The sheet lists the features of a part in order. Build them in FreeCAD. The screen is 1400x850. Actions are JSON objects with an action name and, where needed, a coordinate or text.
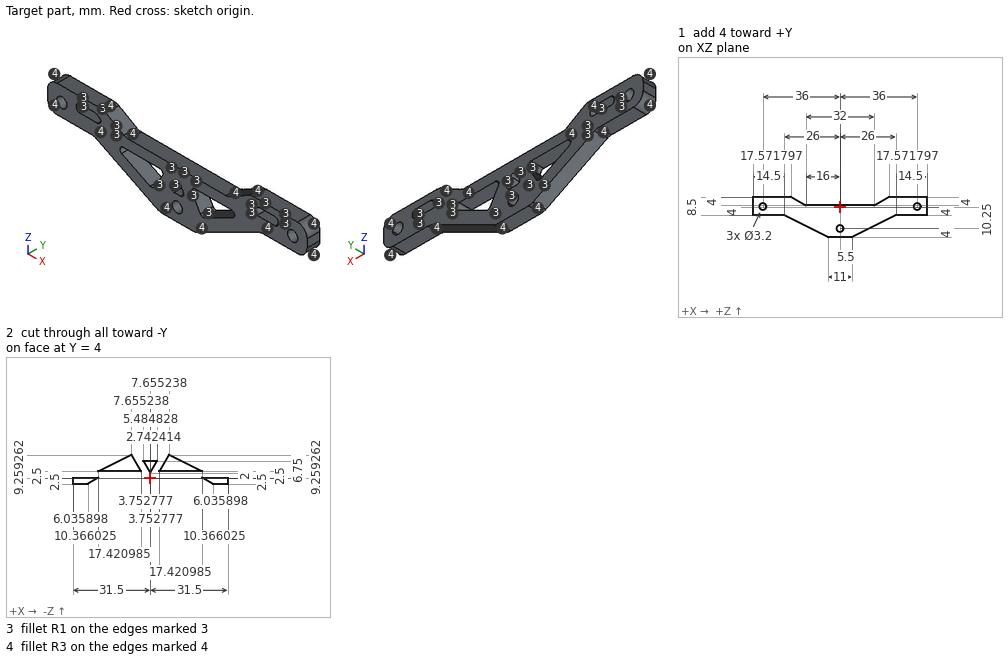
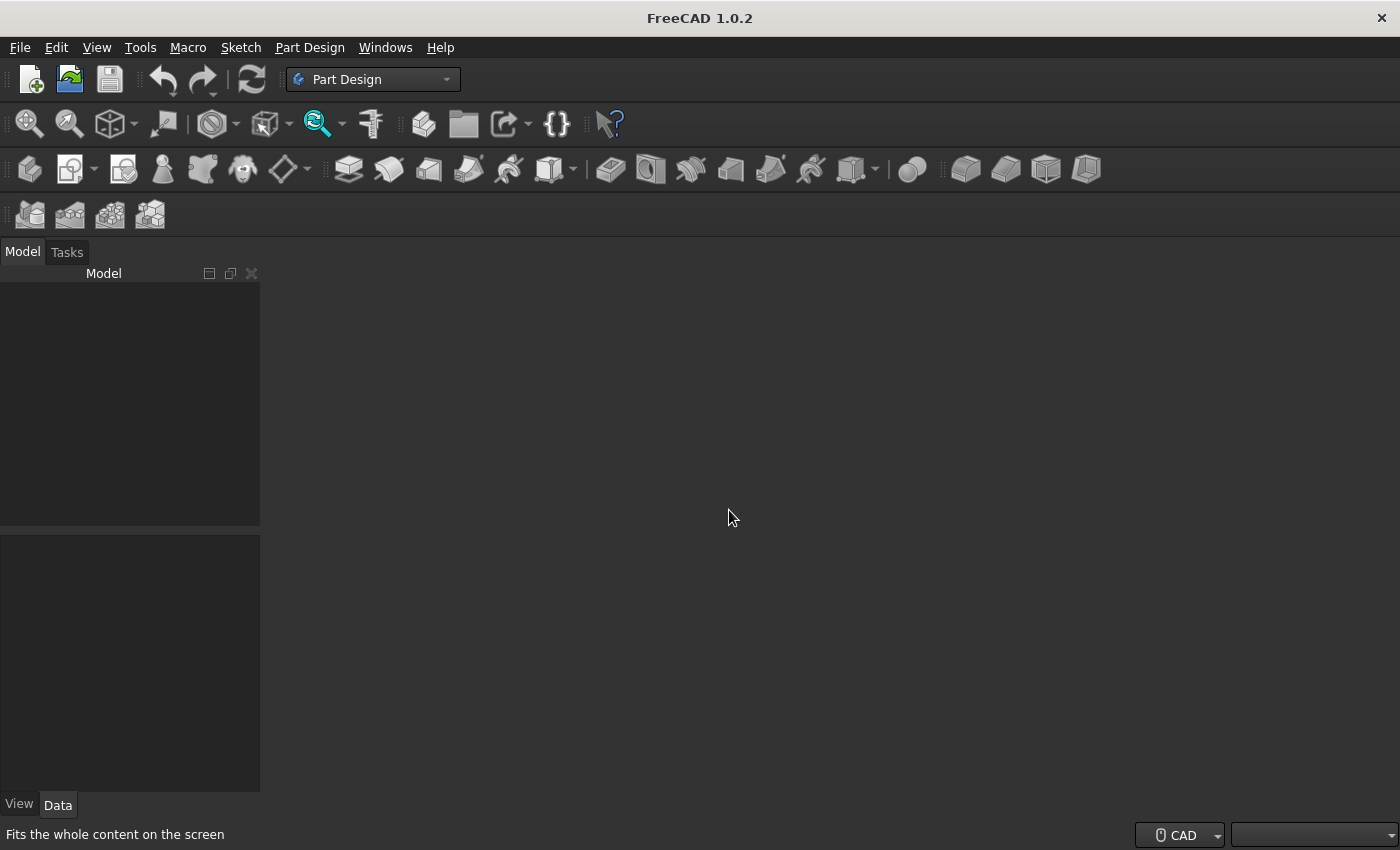
{"action": "left_click", "coordinate": [30, 80]}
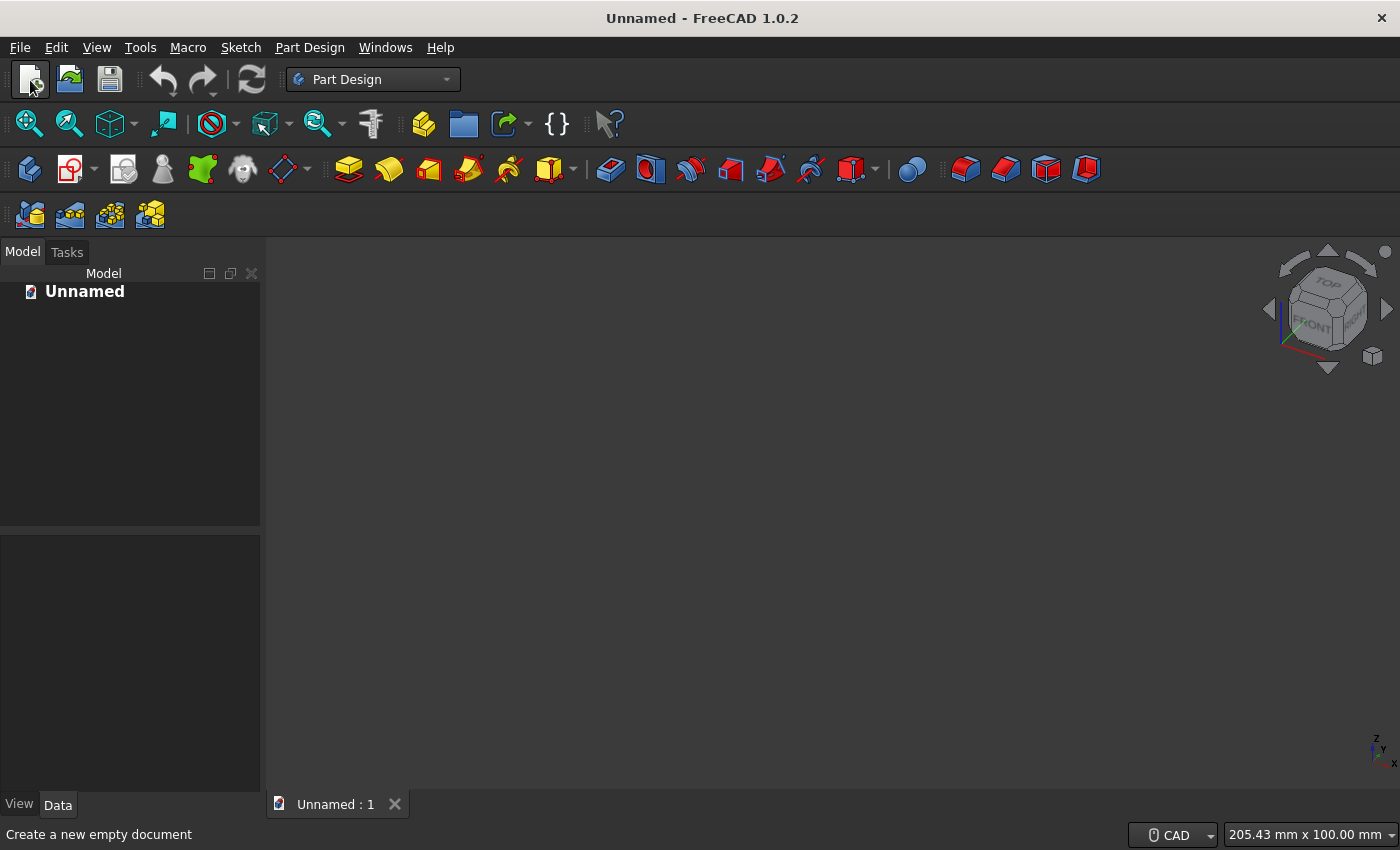
{"action": "left_click", "coordinate": [70, 170]}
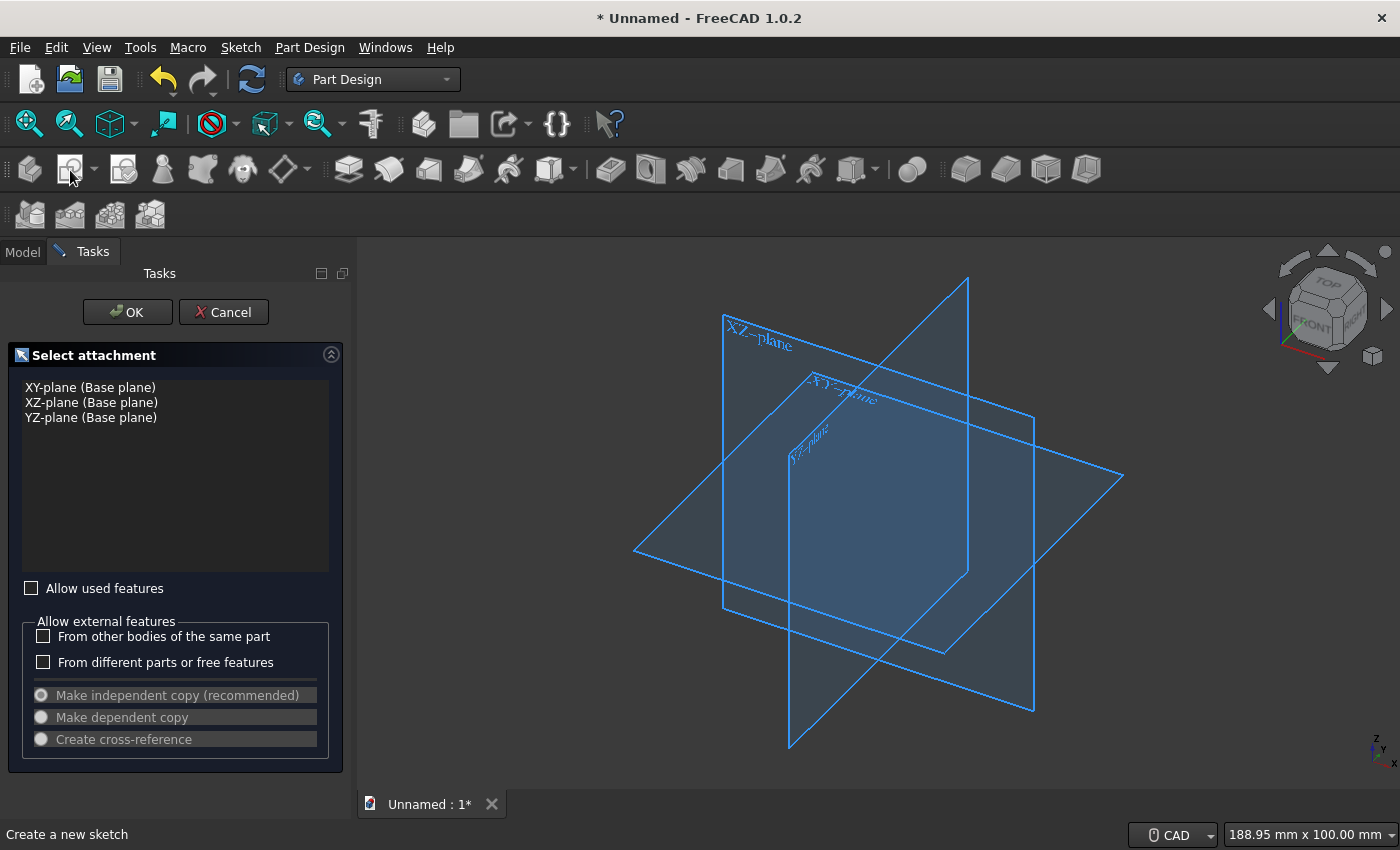
{"action": "left_click", "coordinate": [82, 402]}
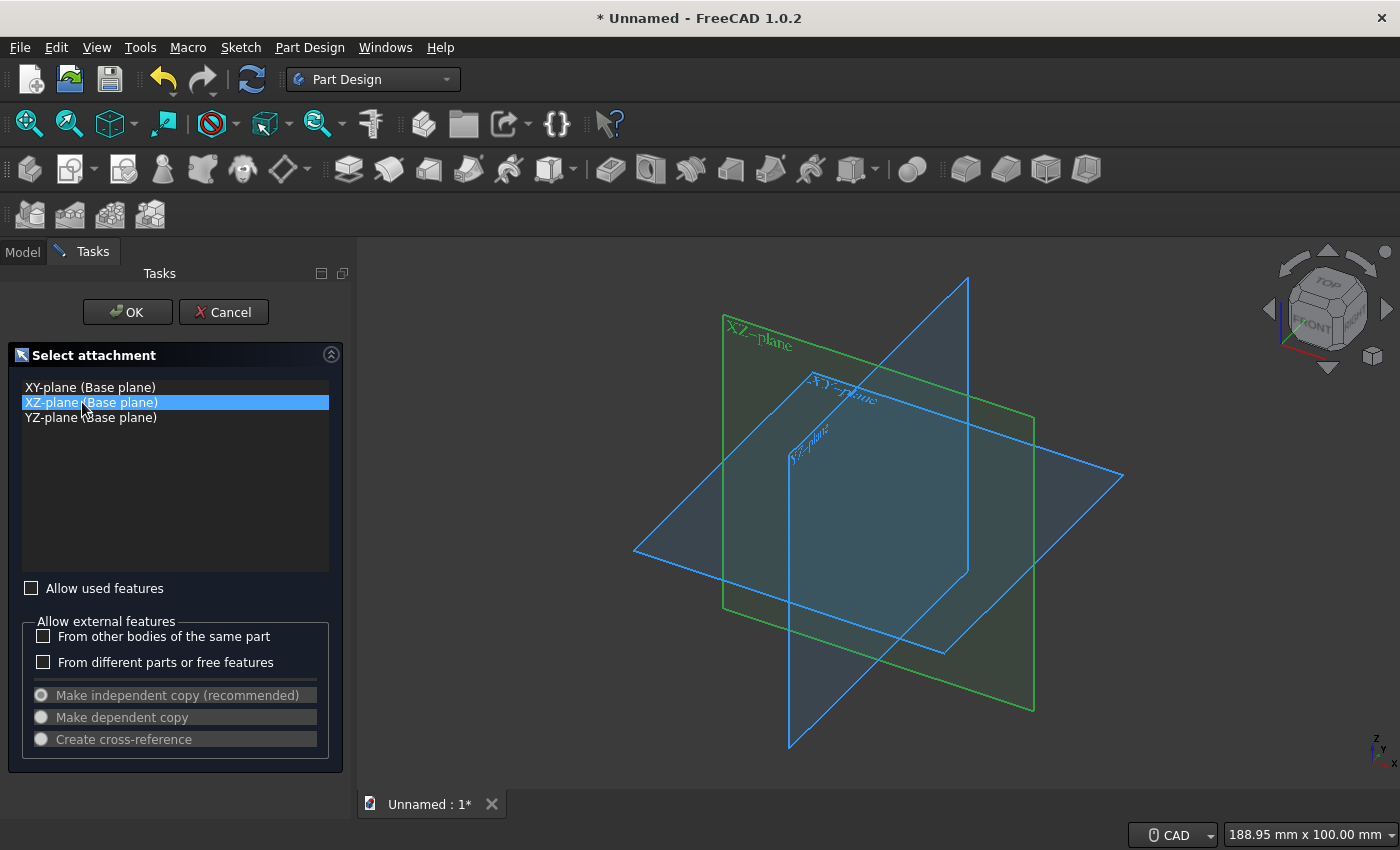
{"action": "left_click", "coordinate": [128, 312]}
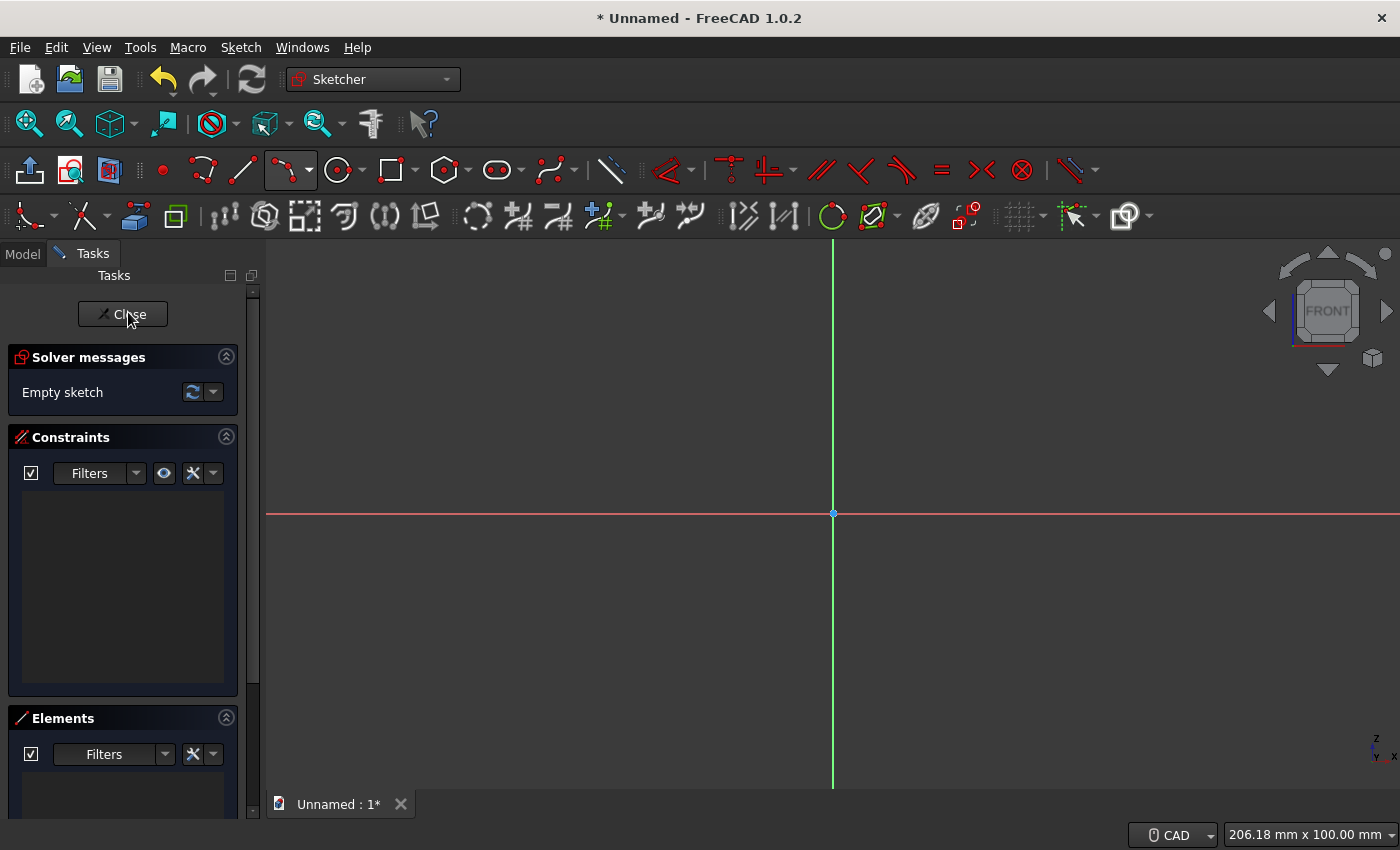
{"action": "scroll", "coordinate": [972, 595], "scroll_direction": "up", "scroll_amount": 2}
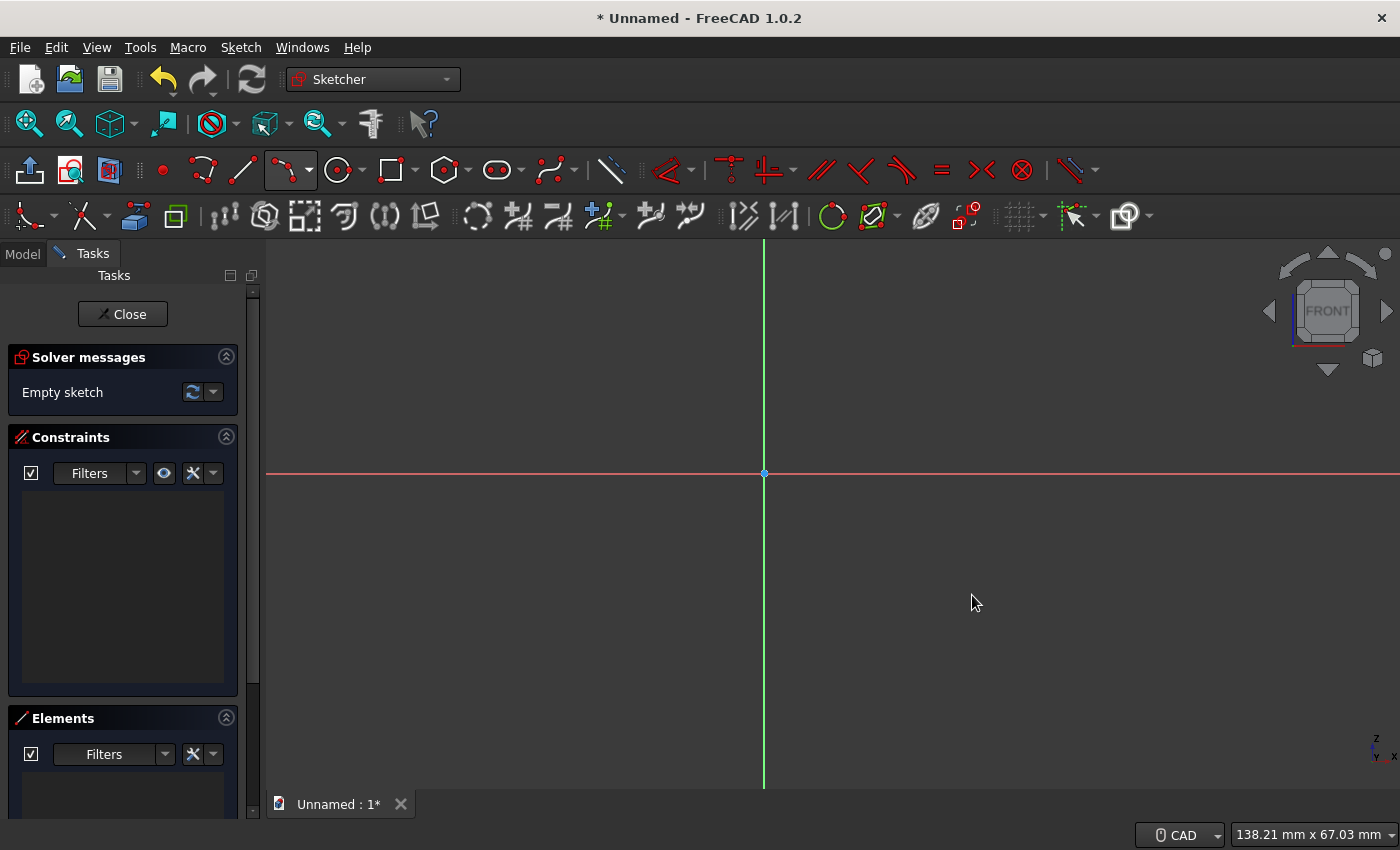
{"action": "left_click", "coordinate": [204, 170]}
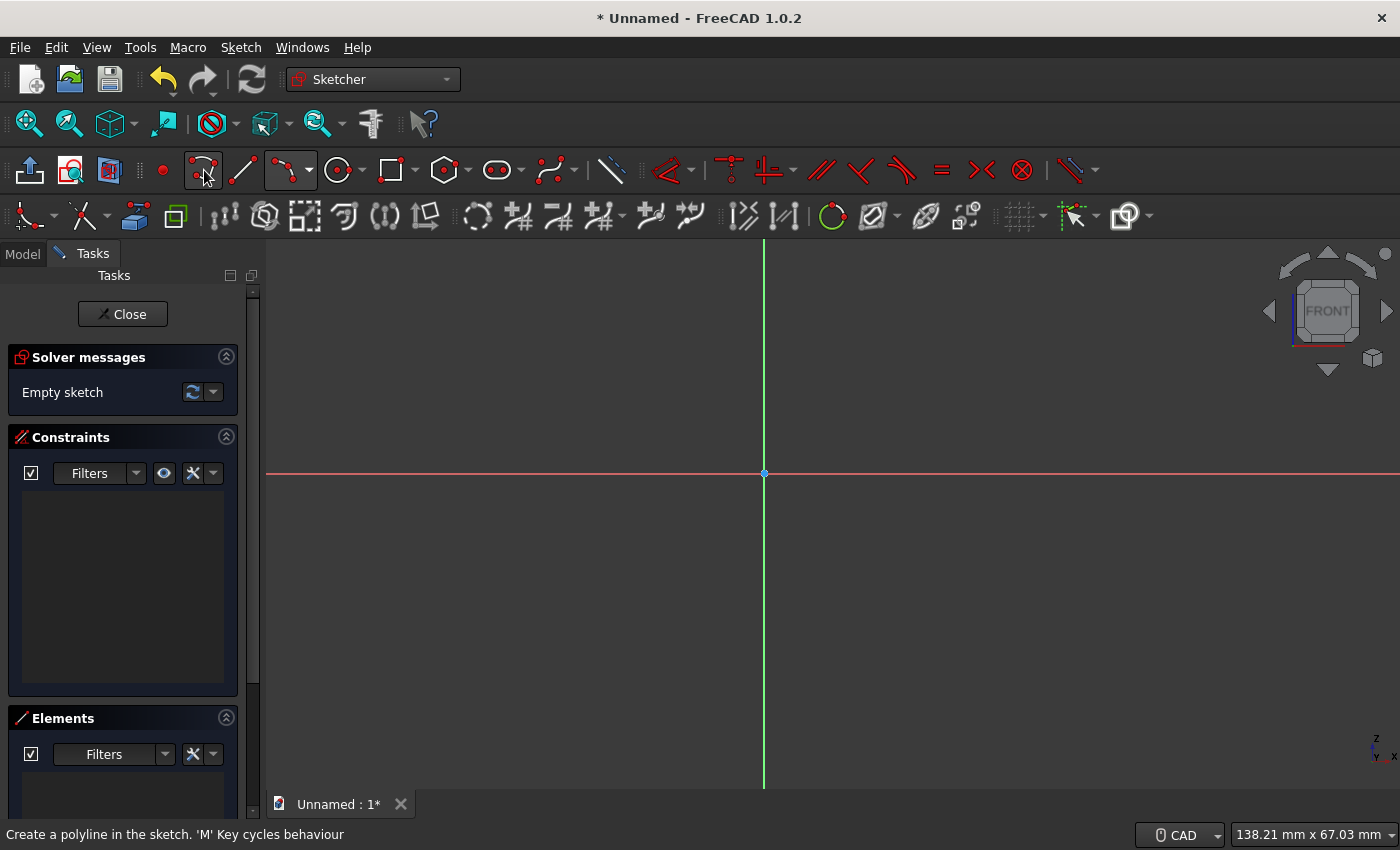
{"action": "left_click", "coordinate": [809, 591]}
{"action": "left_click", "coordinate": [719, 591]}
{"action": "left_click", "coordinate": [551, 507]}
{"action": "left_click", "coordinate": [432, 507]}
{"action": "left_click", "coordinate": [432, 437]}
{"action": "left_click", "coordinate": [576, 437]}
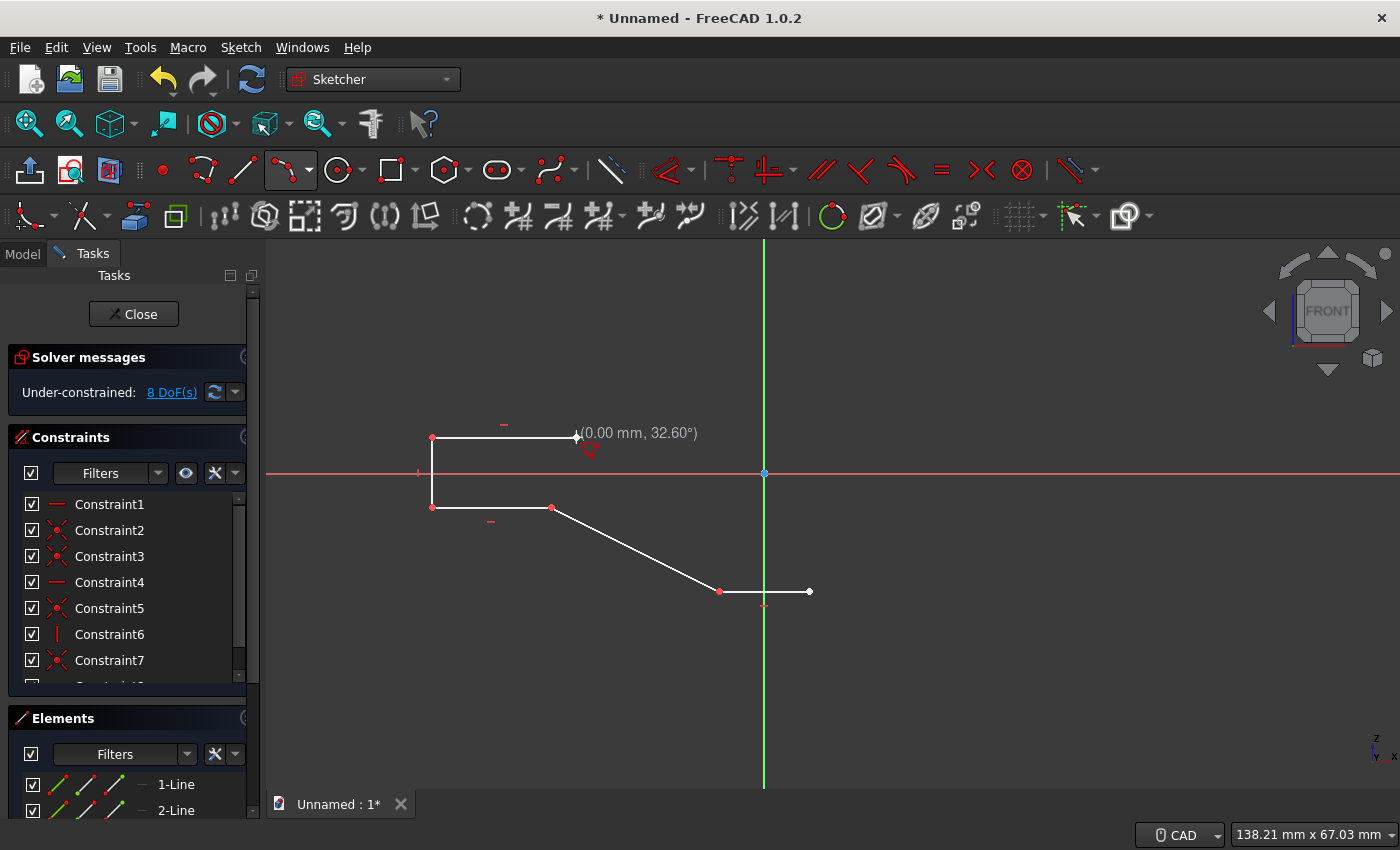
{"action": "scroll", "coordinate": [633, 470], "scroll_direction": "up", "scroll_amount": 7}